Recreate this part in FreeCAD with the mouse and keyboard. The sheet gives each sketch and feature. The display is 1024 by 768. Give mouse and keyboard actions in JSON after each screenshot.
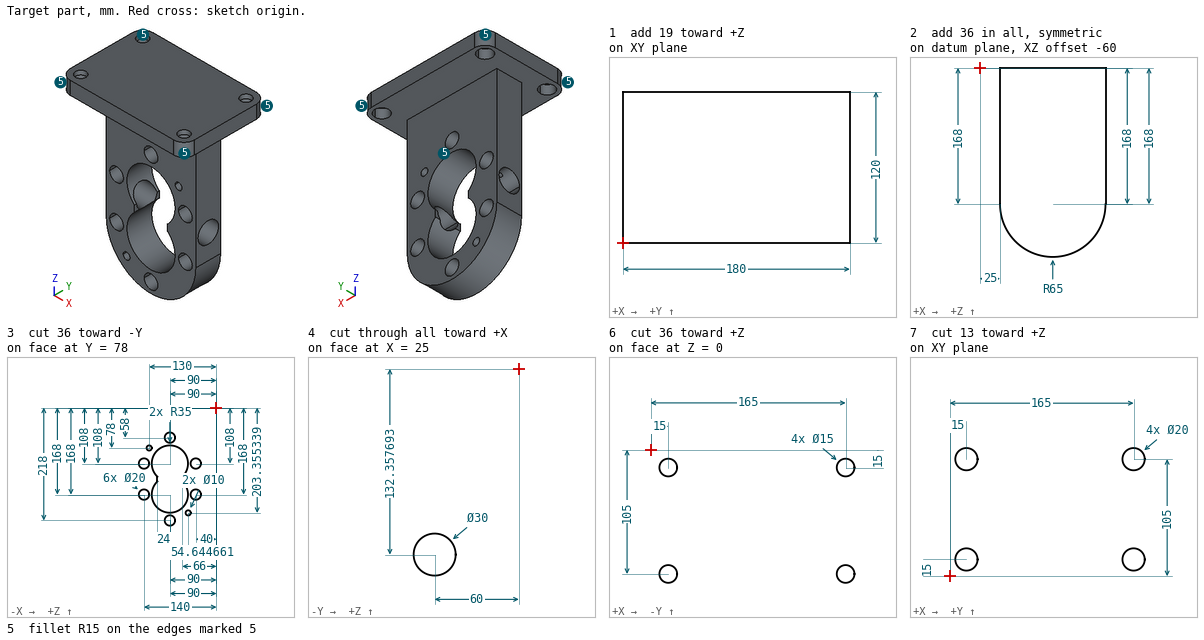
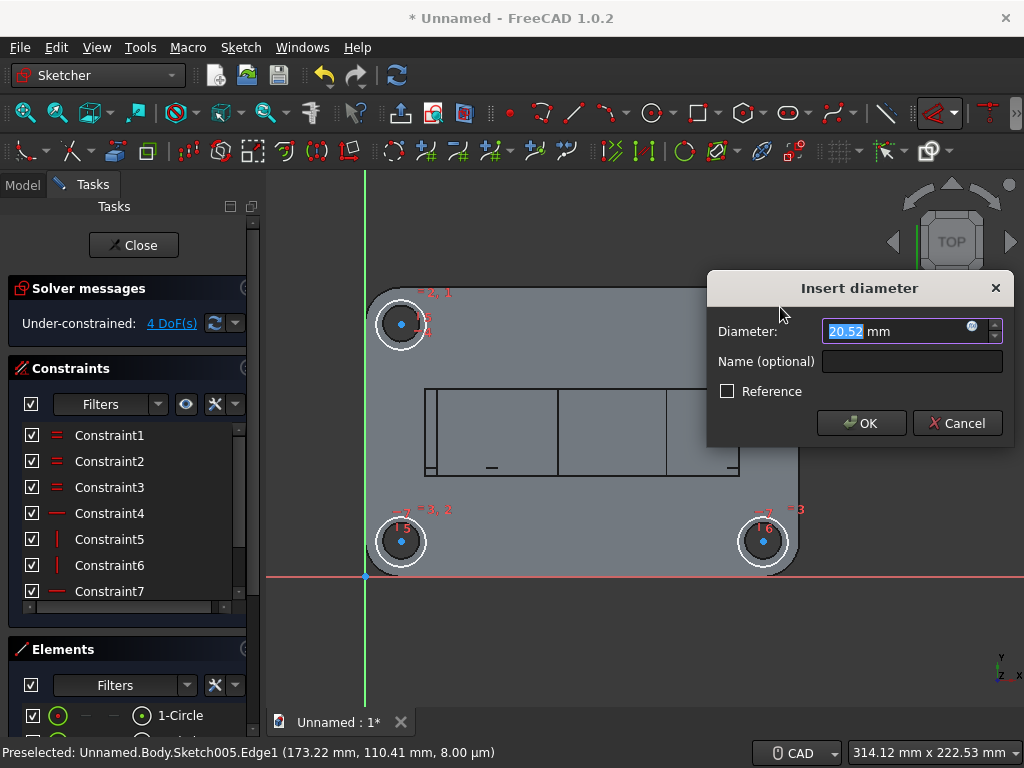
{"action": "type", "text": "20"}
{"action": "key", "text": "Return"}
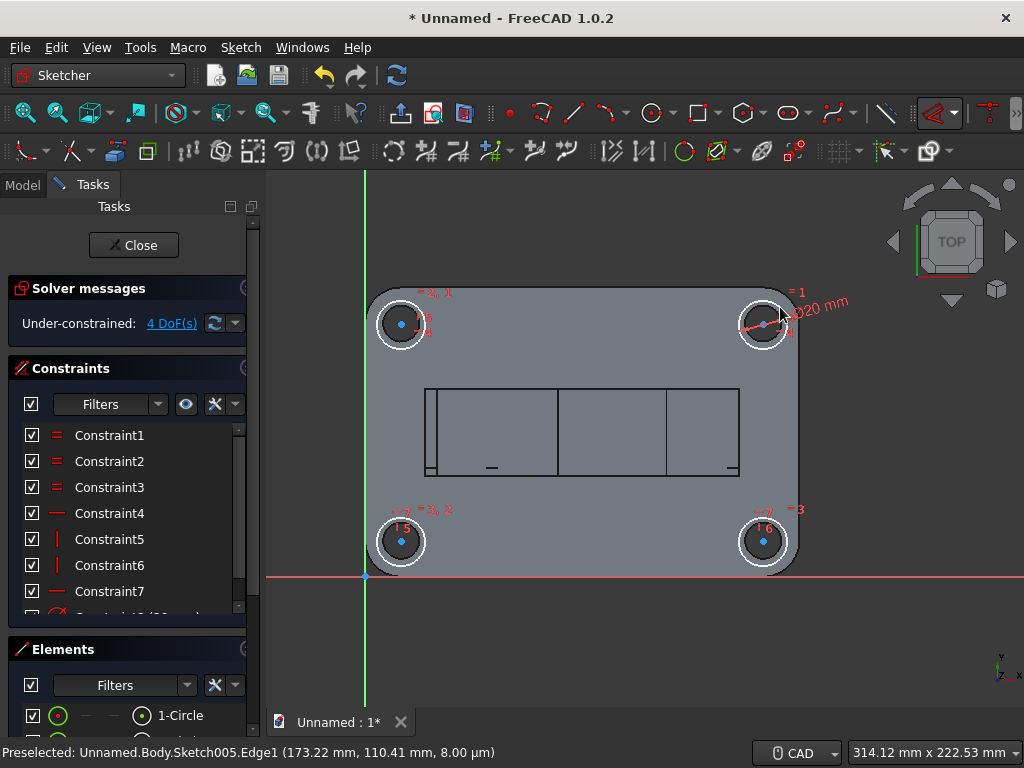
{"action": "left_click", "coordinate": [401, 325]}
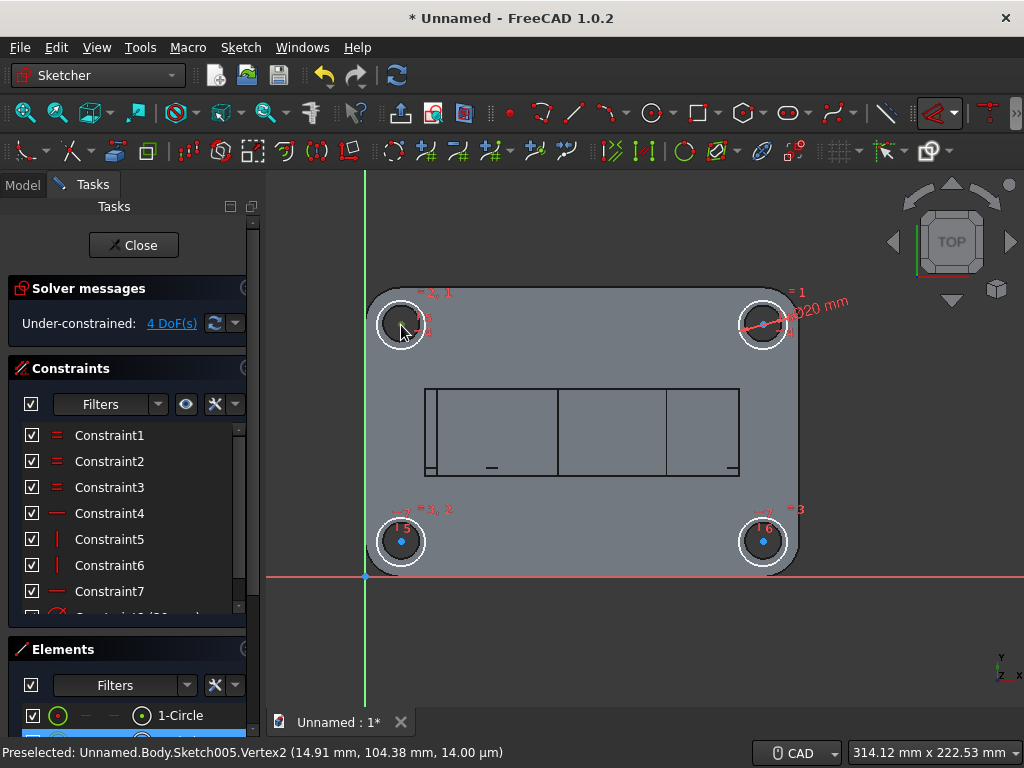
{"action": "left_click", "coordinate": [956, 114]}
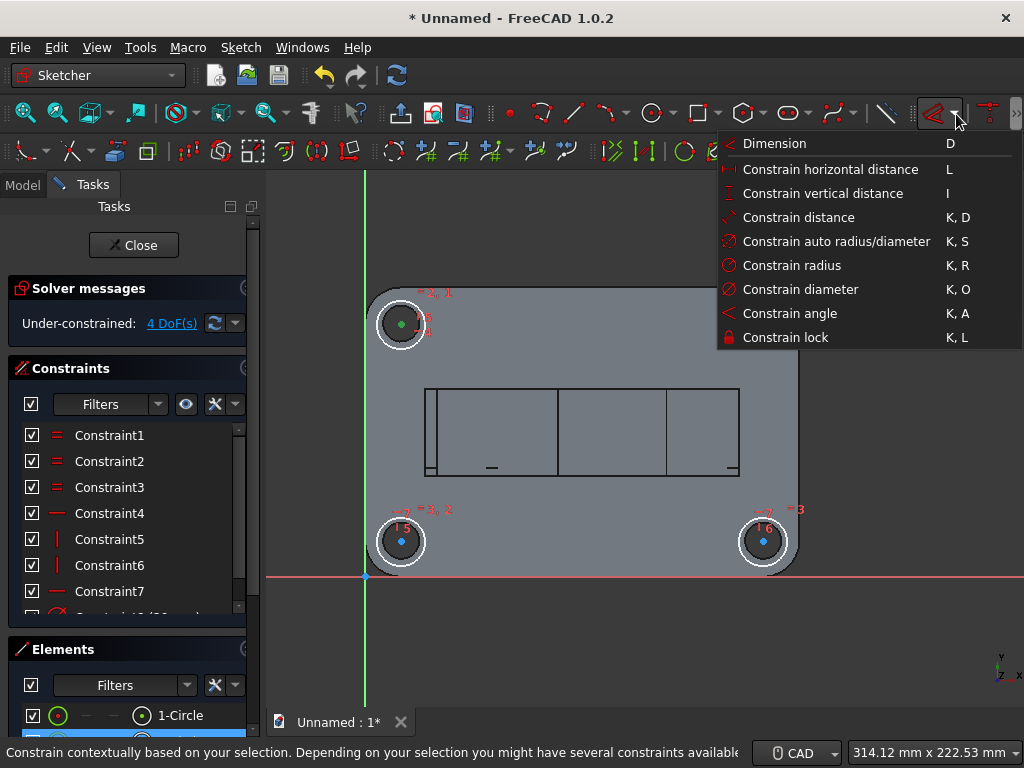
{"action": "left_click", "coordinate": [870, 169]}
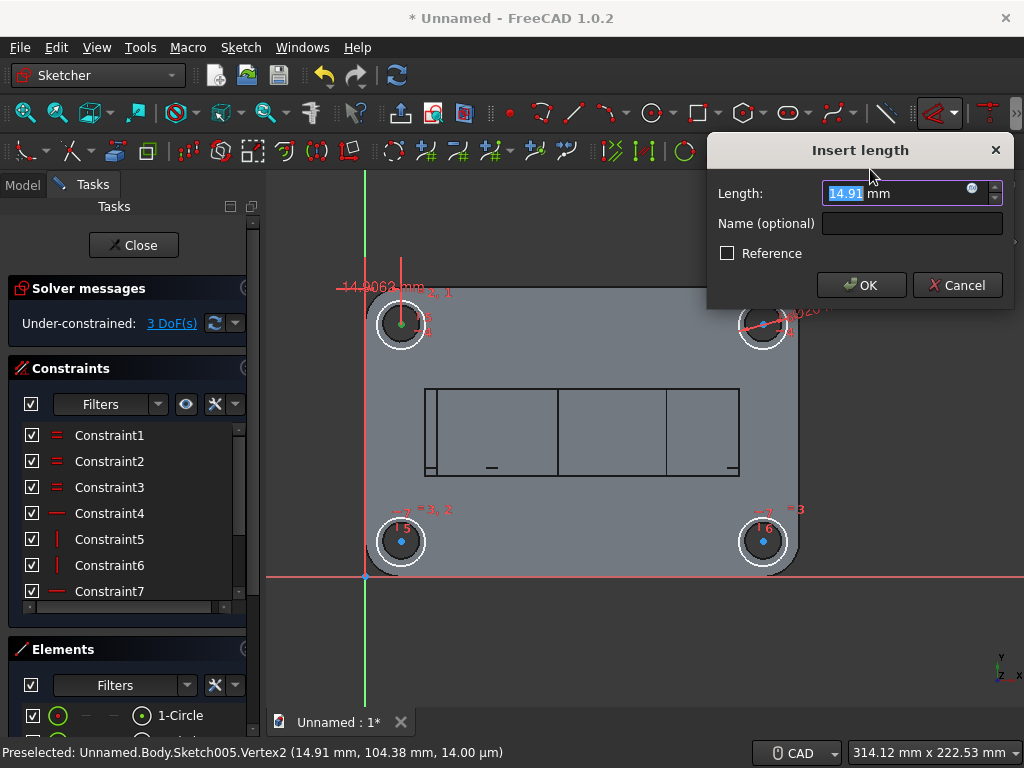
{"action": "type", "text": "15"}
{"action": "key", "text": "Return"}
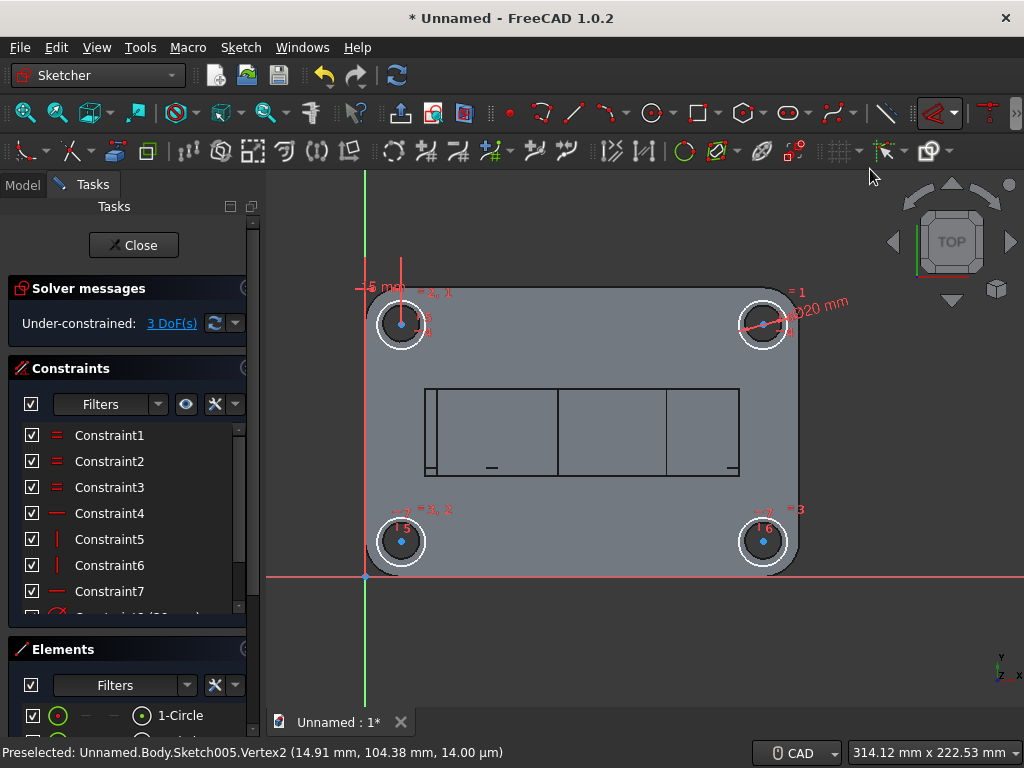
{"action": "left_click", "coordinate": [401, 542]}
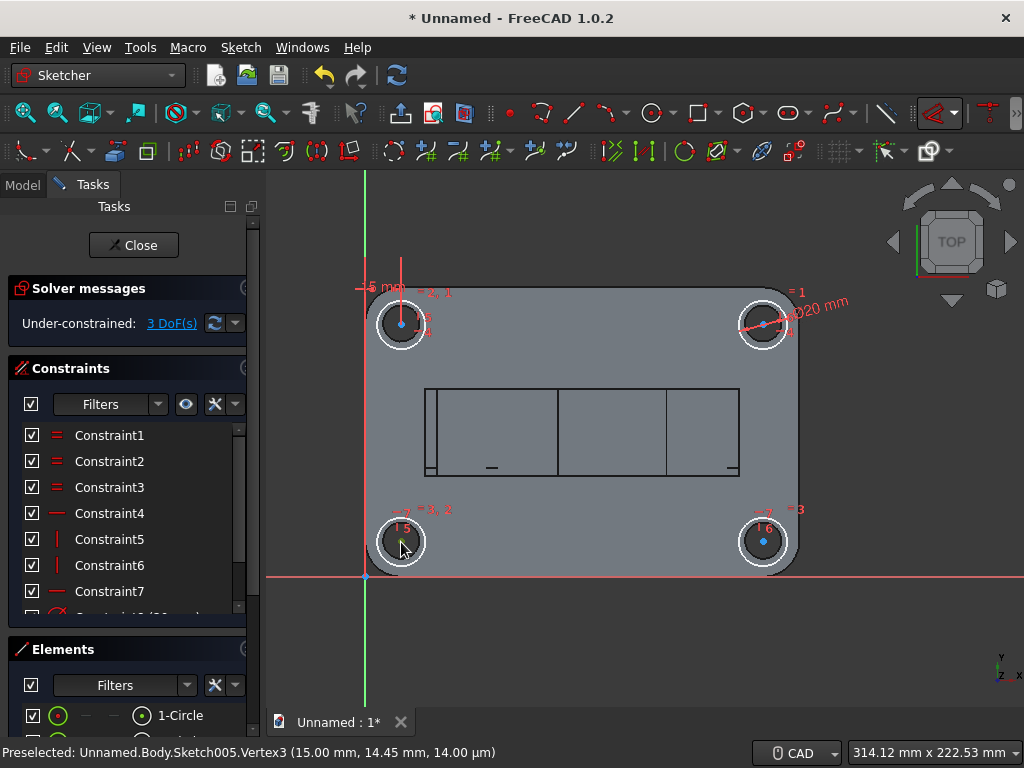
{"action": "key", "text": "i"}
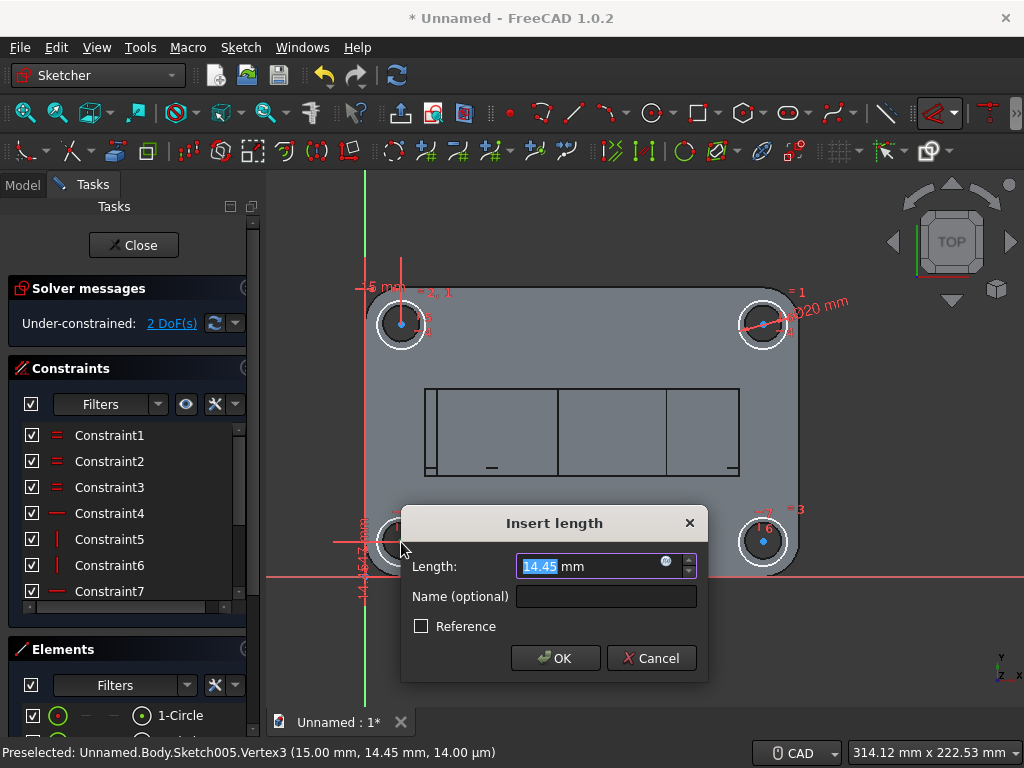
{"action": "type", "text": "15"}
{"action": "key", "text": "Return"}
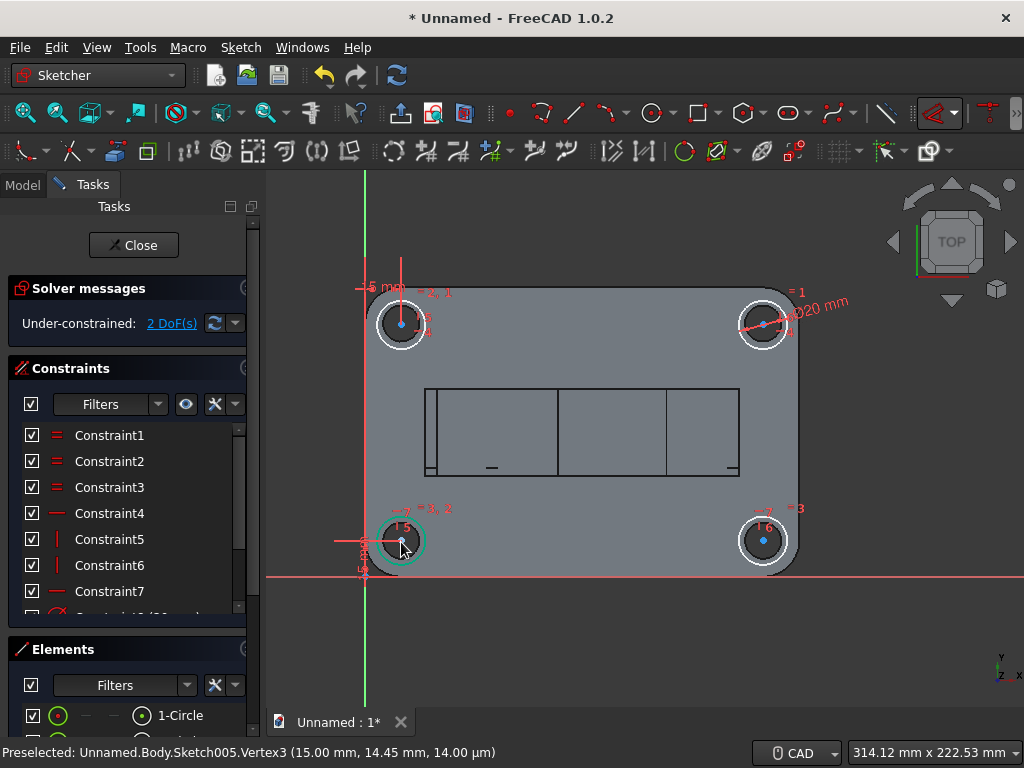
{"action": "left_click", "coordinate": [763, 325]}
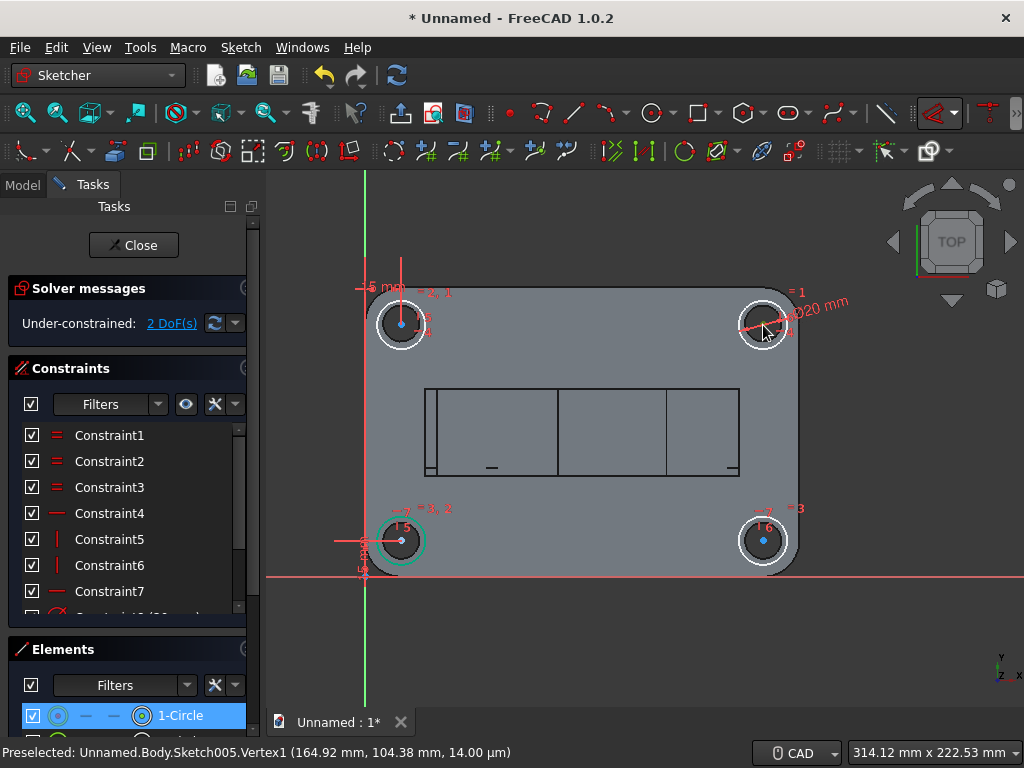
{"action": "left_click", "coordinate": [956, 114]}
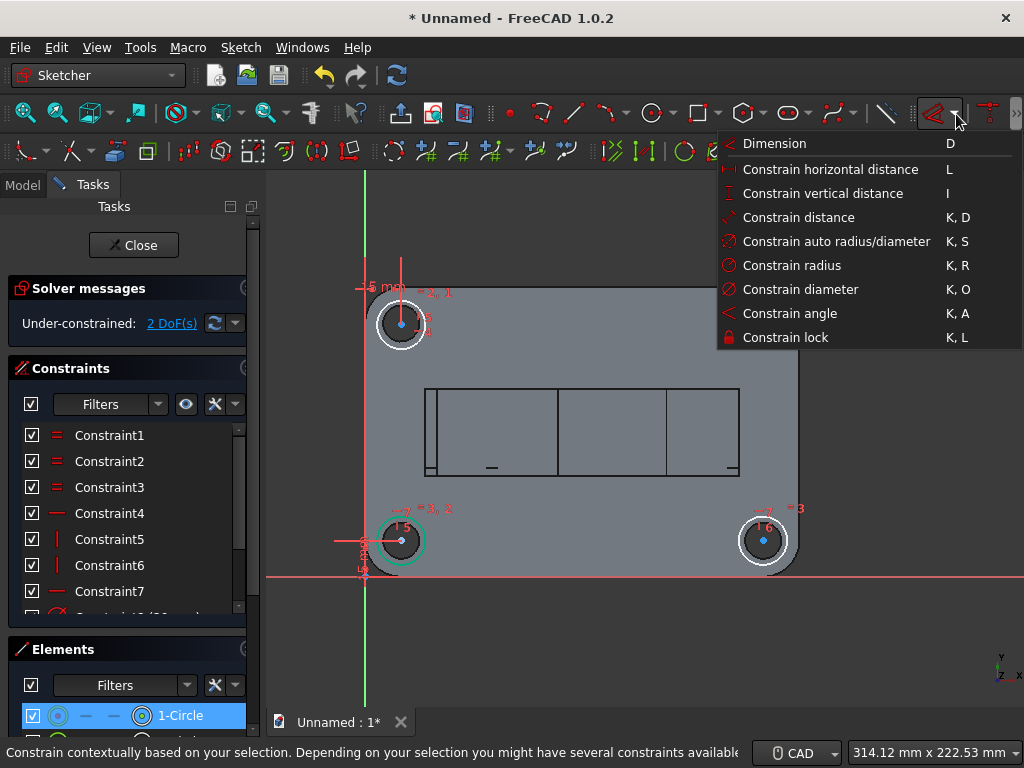
{"action": "left_click", "coordinate": [870, 169]}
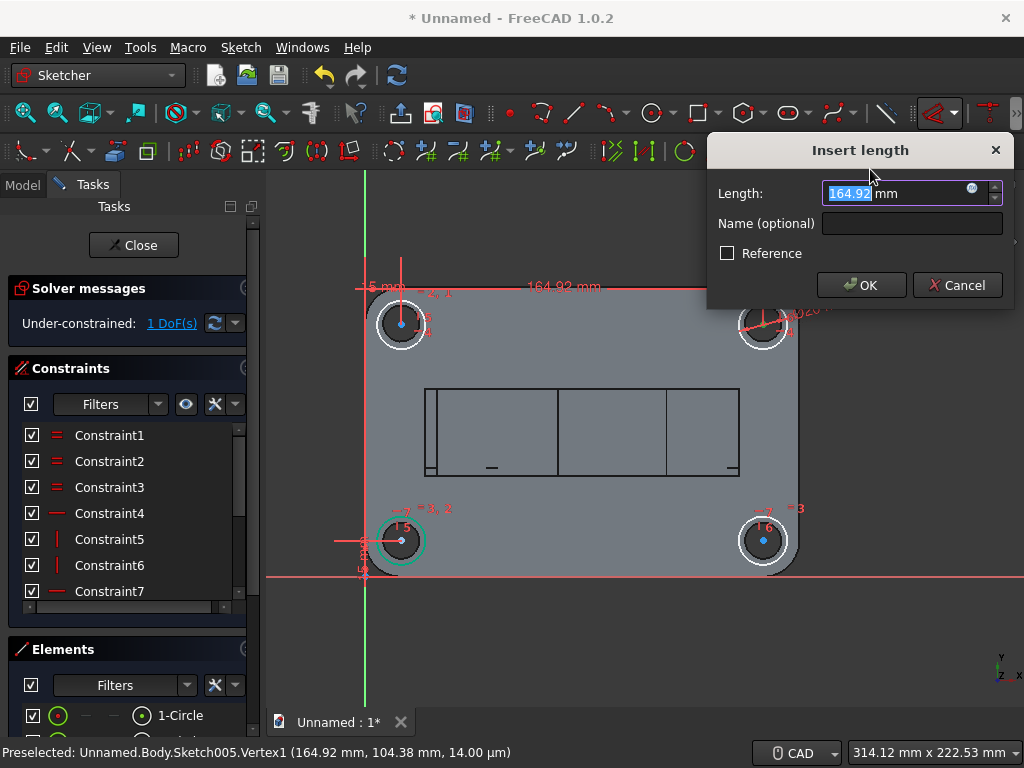
{"action": "type", "text": "165"}
{"action": "key", "text": "Return"}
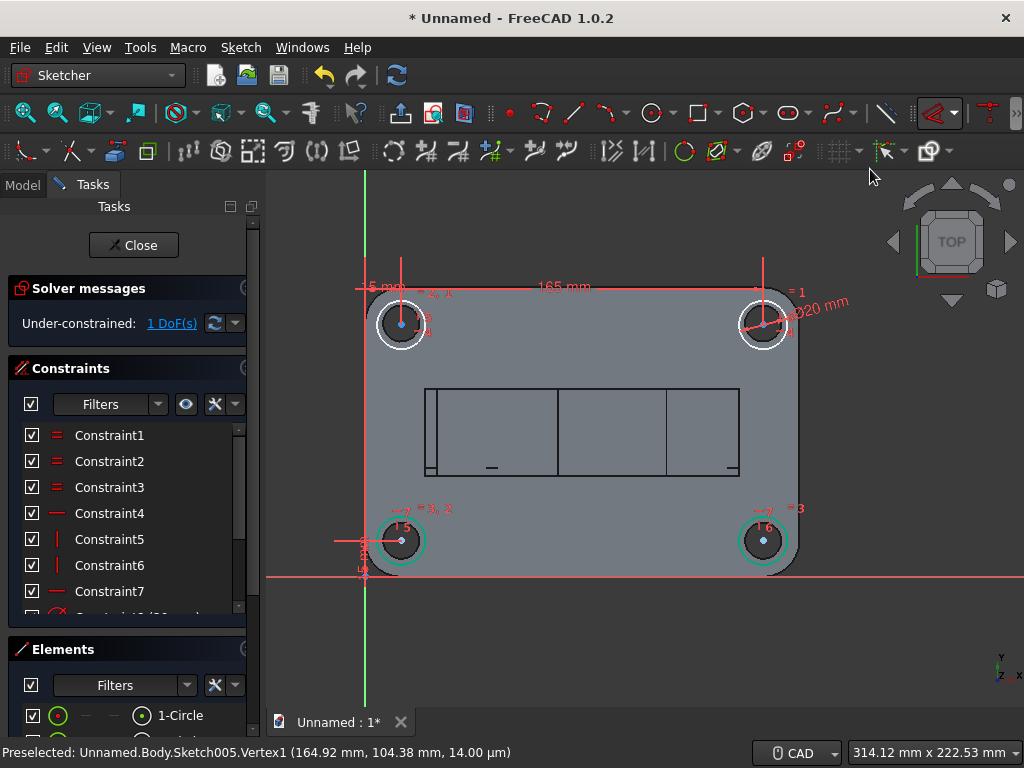
{"action": "left_click", "coordinate": [763, 325]}